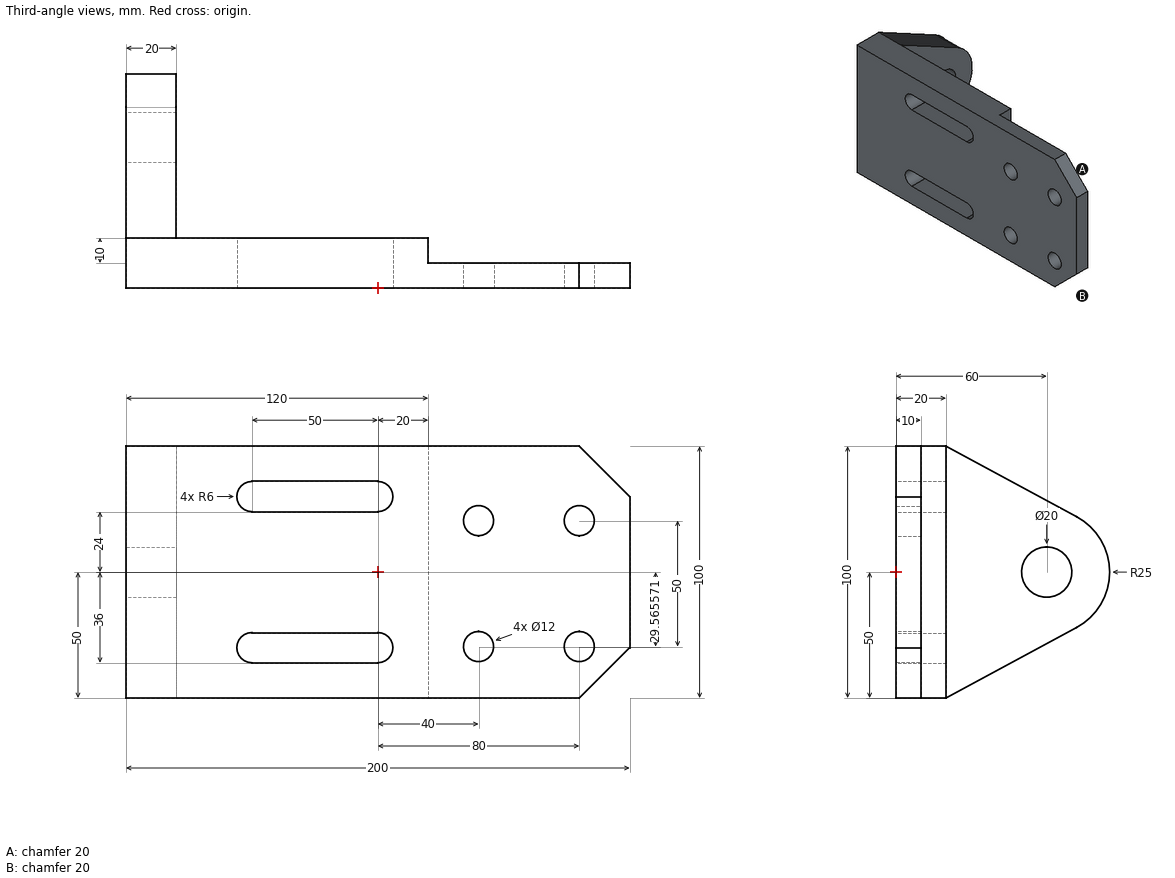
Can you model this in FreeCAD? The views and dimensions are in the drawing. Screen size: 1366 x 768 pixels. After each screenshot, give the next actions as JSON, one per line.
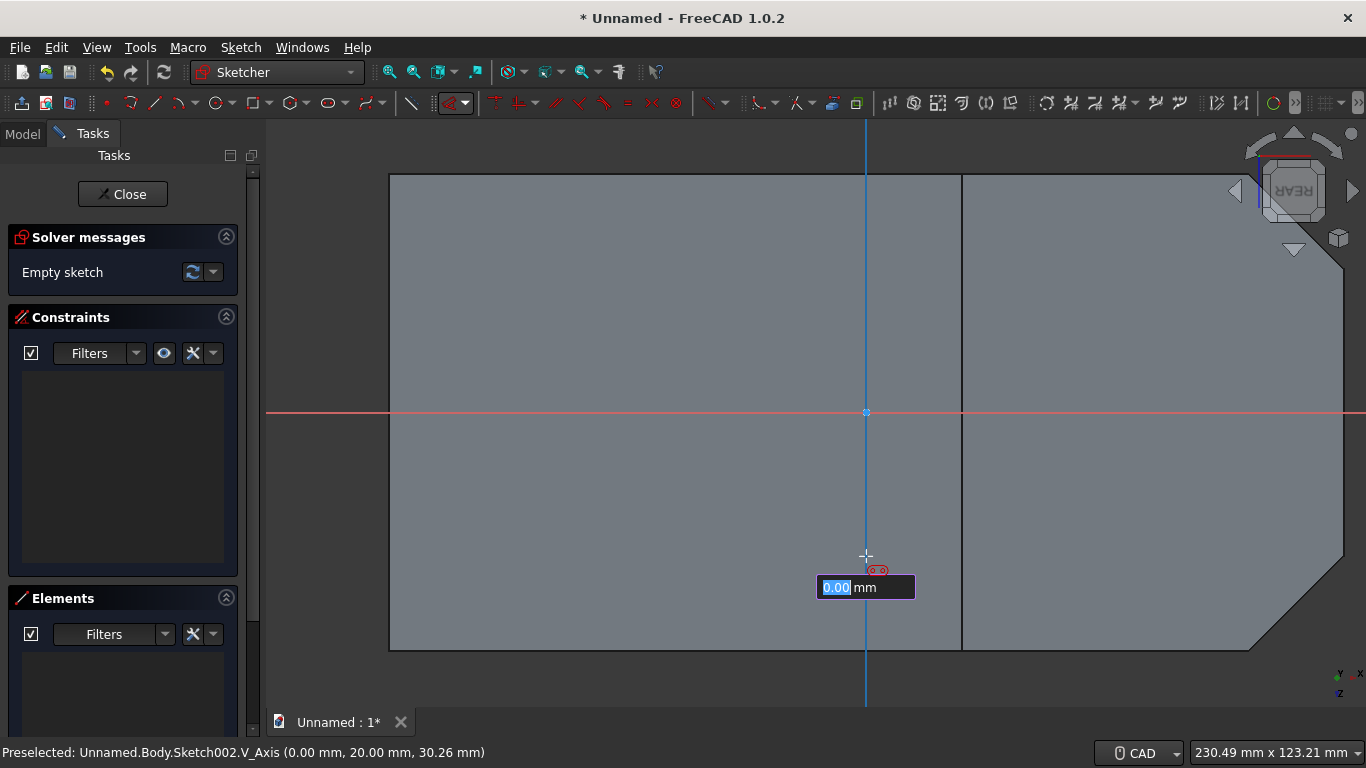
{"action": "left_click", "coordinate": [747, 527]}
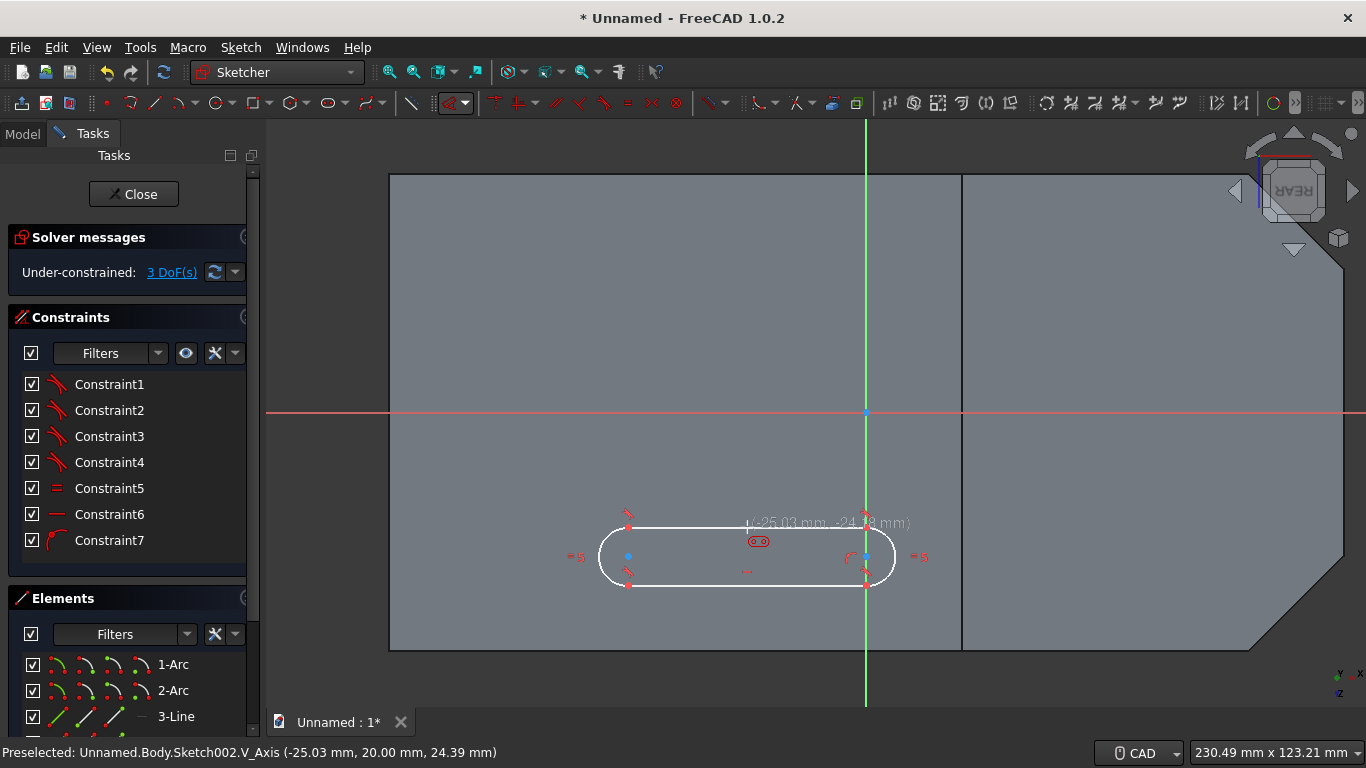
{"action": "left_click", "coordinate": [628, 269]}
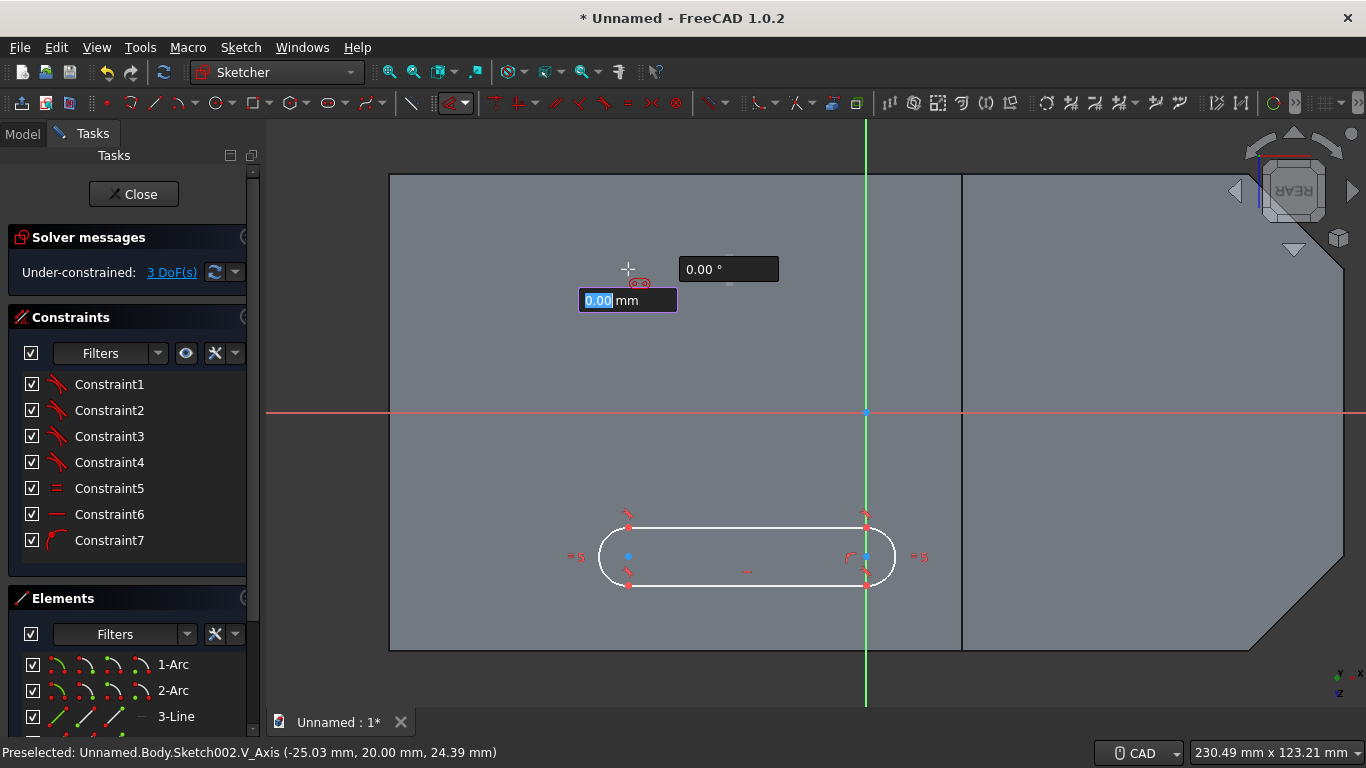
{"action": "left_click", "coordinate": [866, 269]}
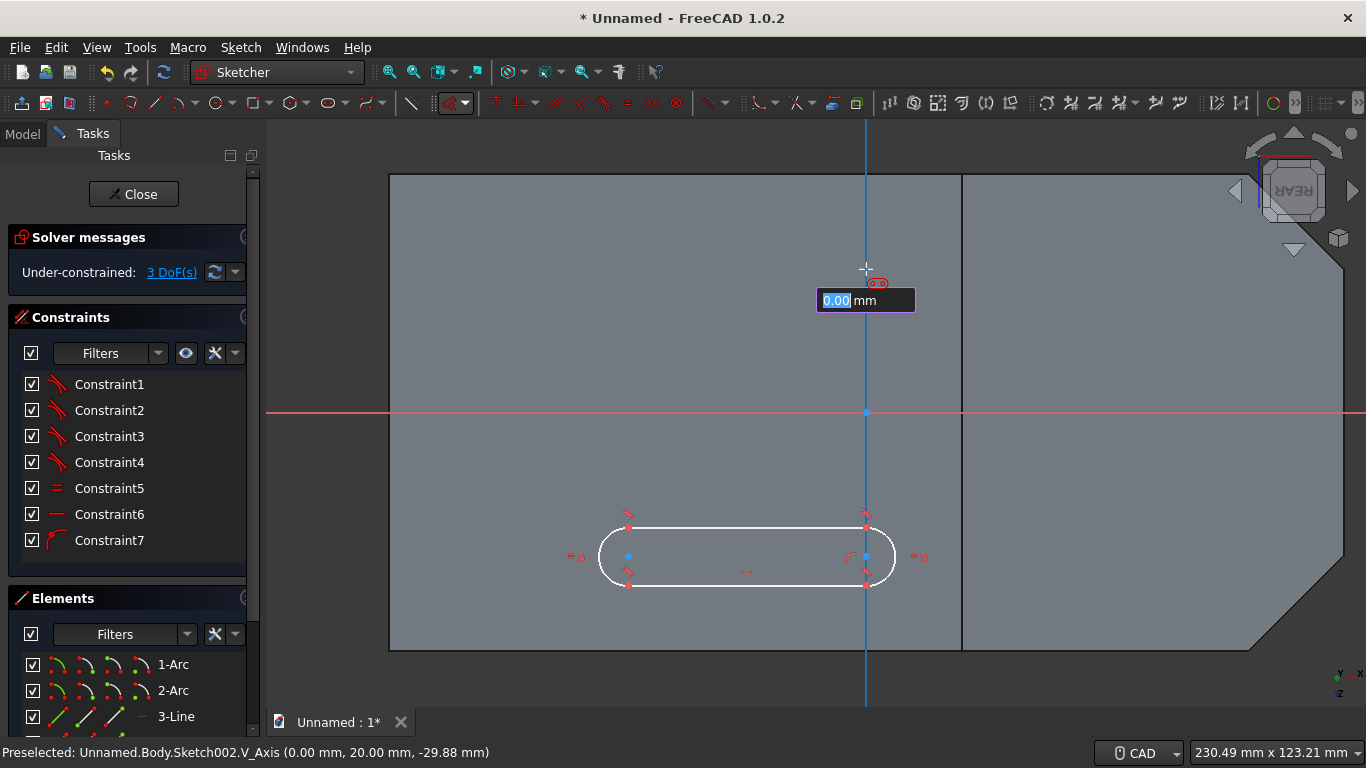
{"action": "left_click", "coordinate": [747, 298]}
{"action": "key", "text": "Escape"}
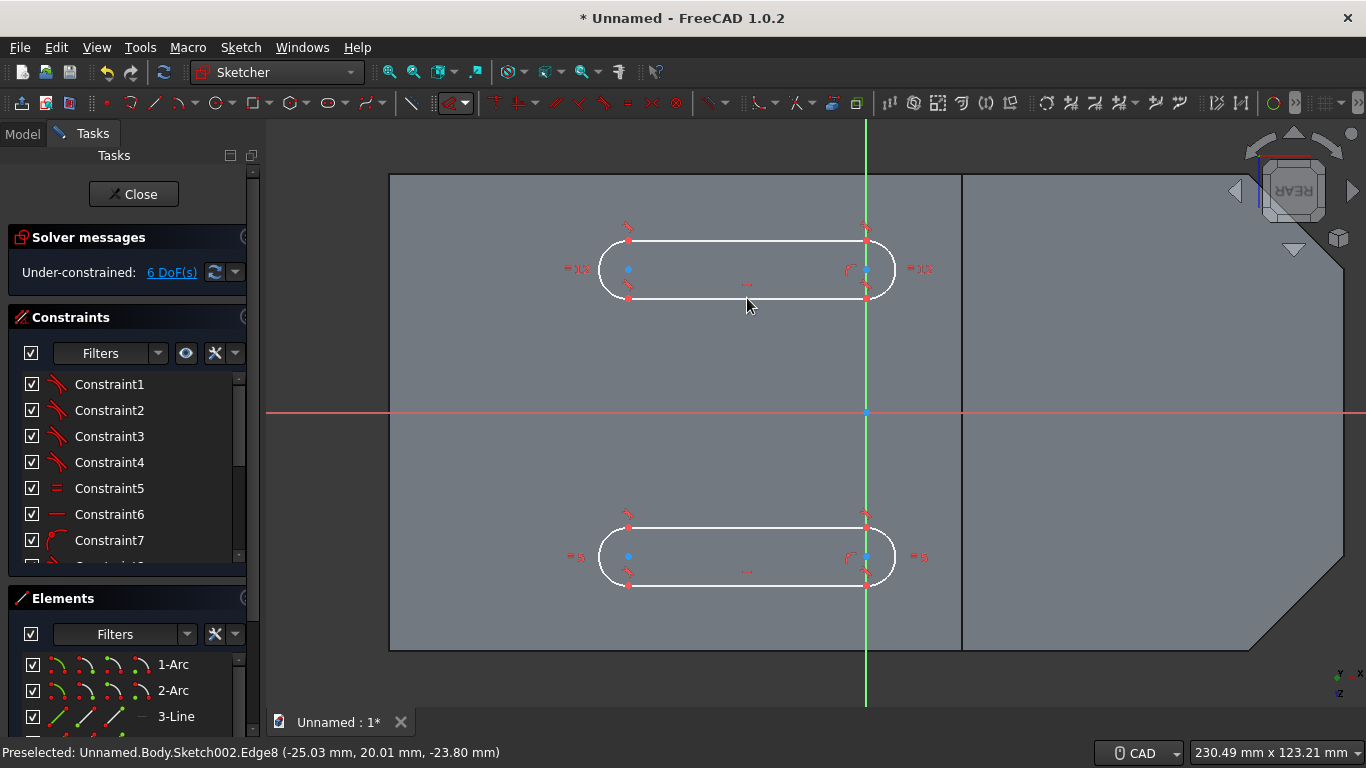
{"action": "left_click", "coordinate": [605, 540]}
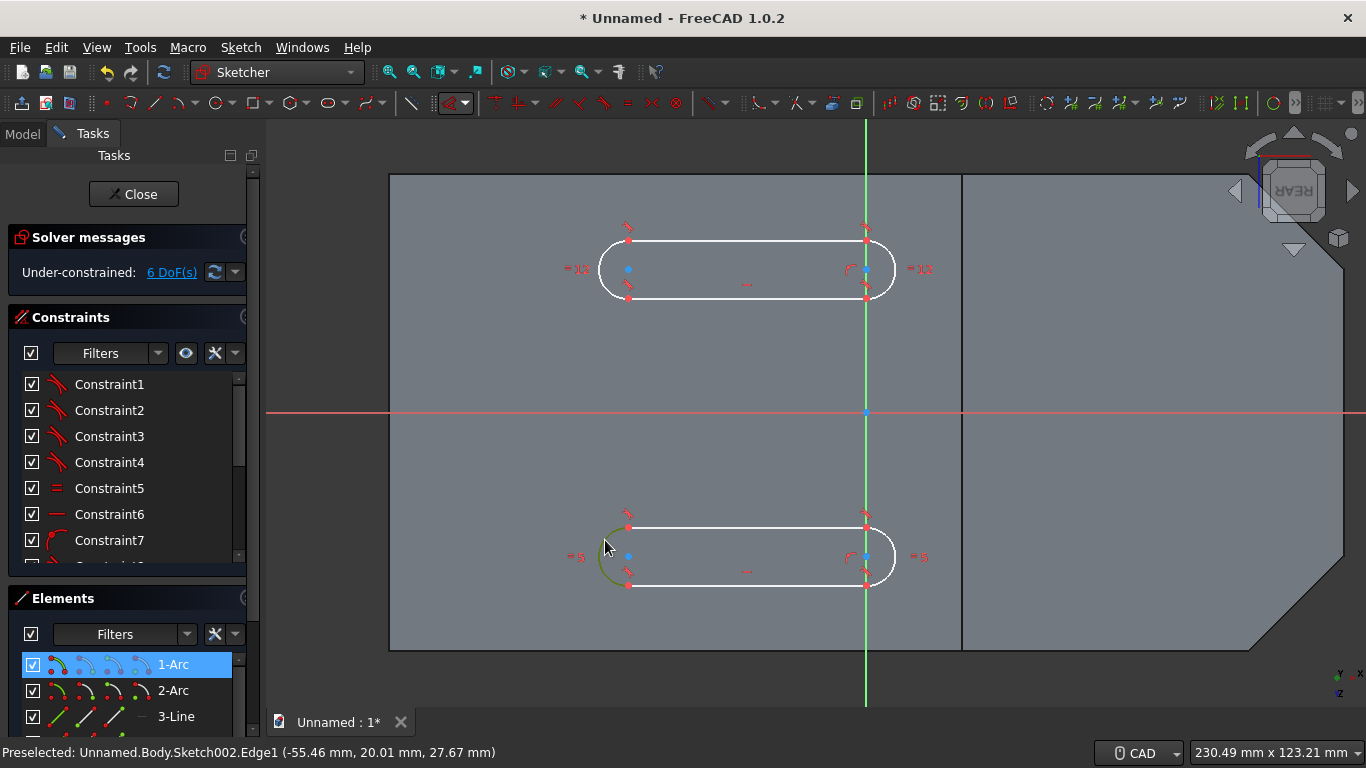
{"action": "left_click", "coordinate": [605, 253]}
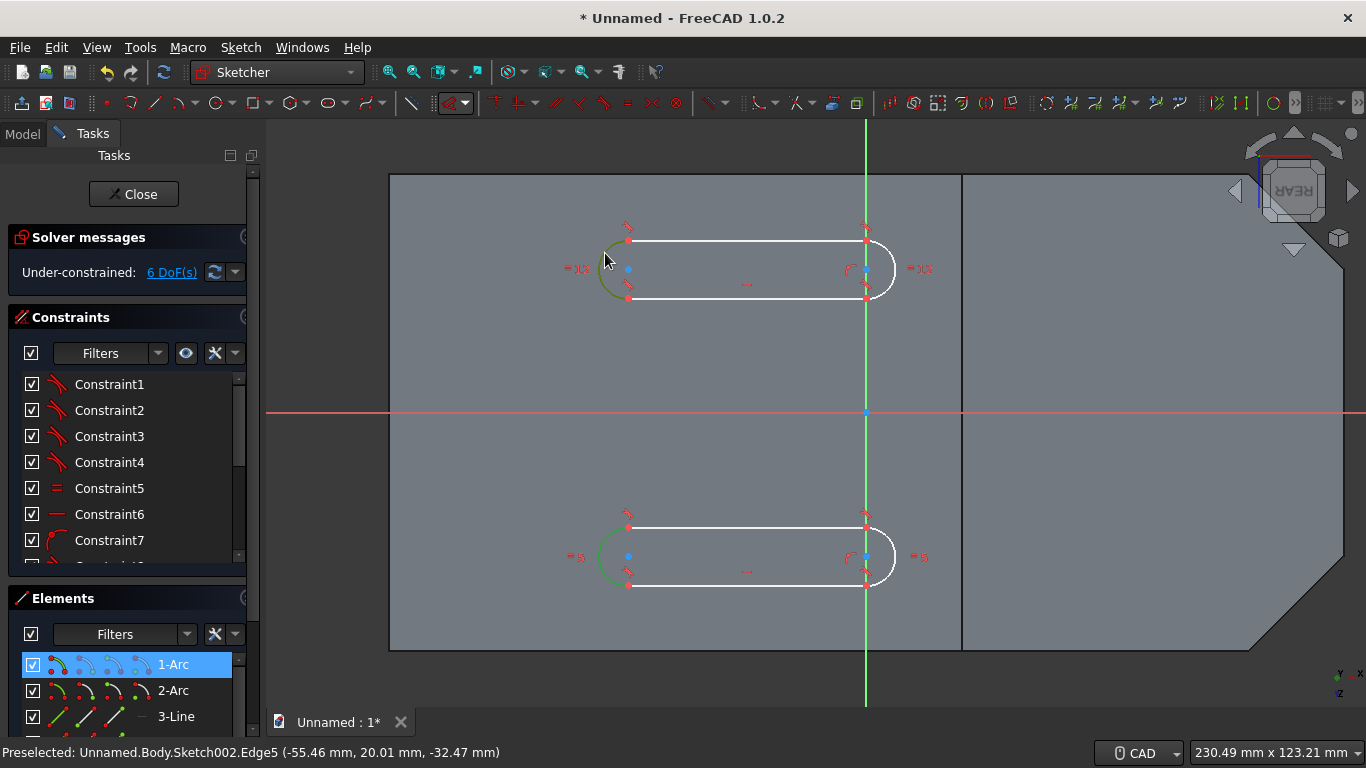
{"action": "left_click", "coordinate": [628, 104]}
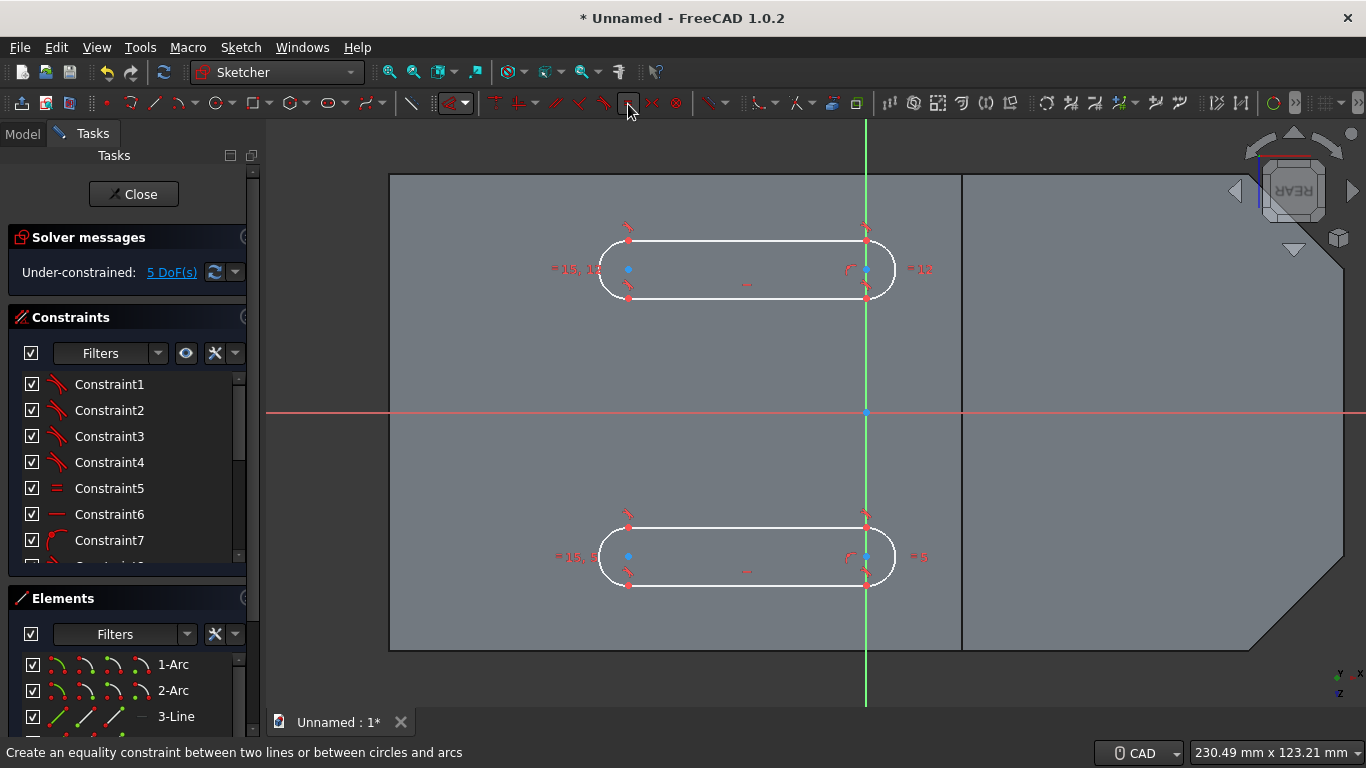
{"action": "scroll", "coordinate": [605, 540], "scroll_direction": "up", "scroll_amount": 2}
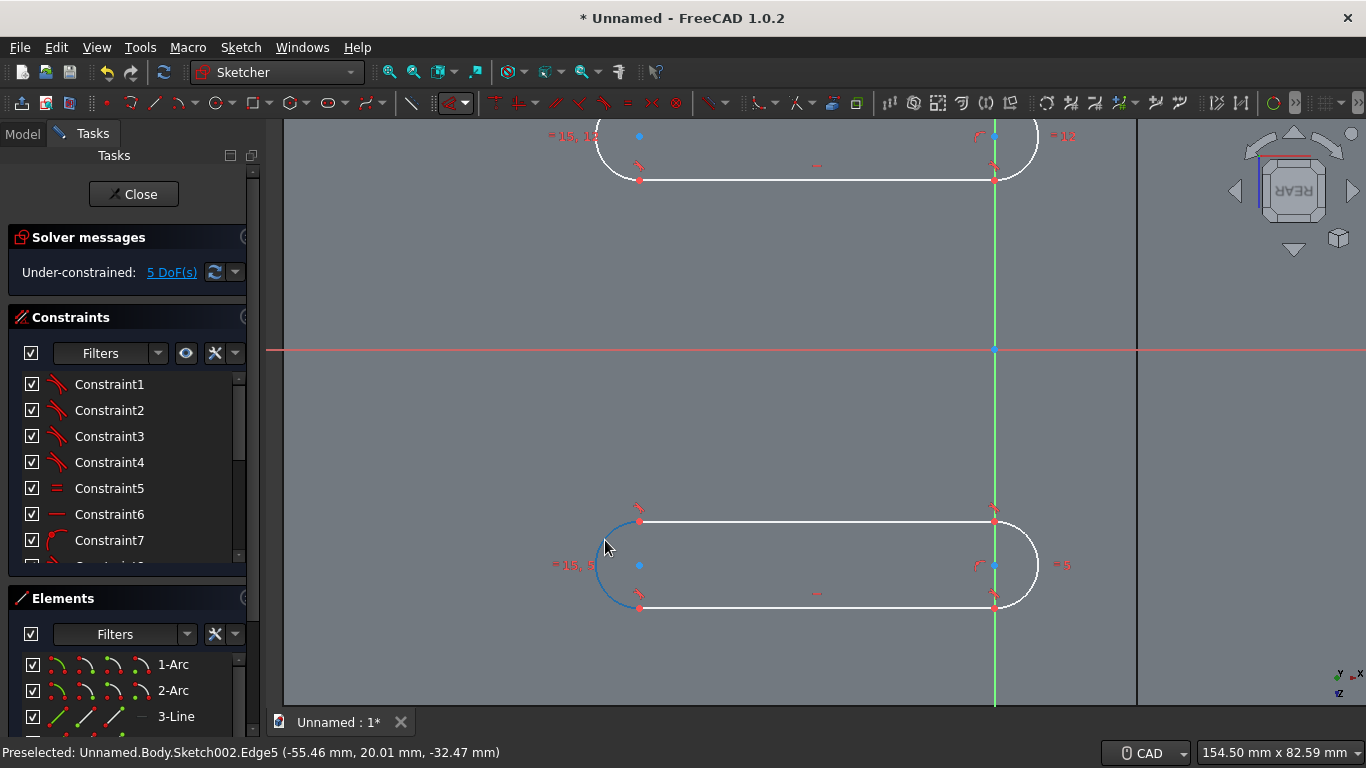
{"action": "left_click", "coordinate": [604, 540]}